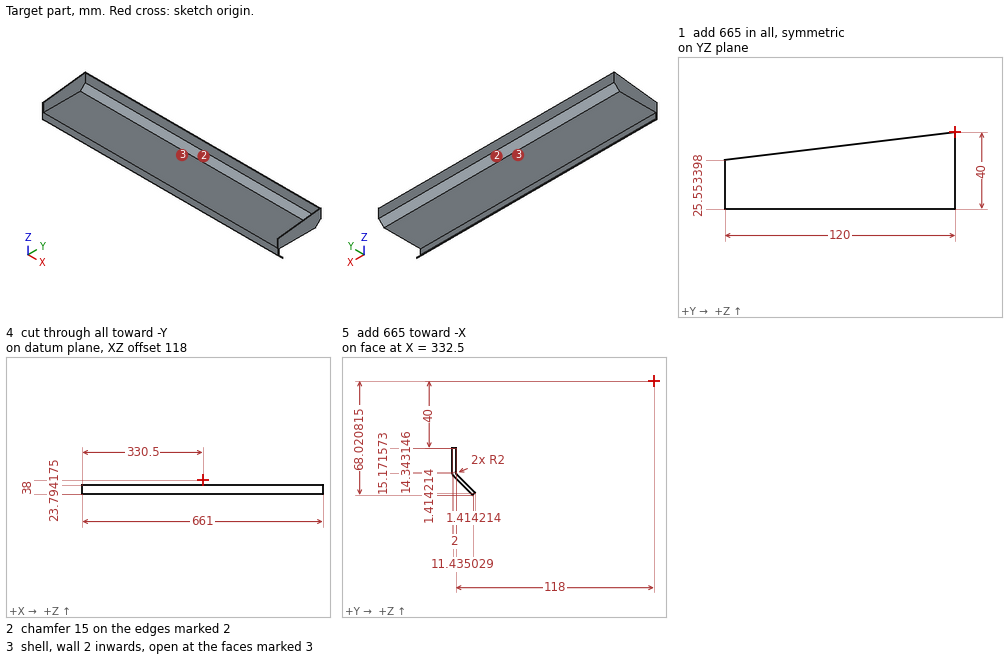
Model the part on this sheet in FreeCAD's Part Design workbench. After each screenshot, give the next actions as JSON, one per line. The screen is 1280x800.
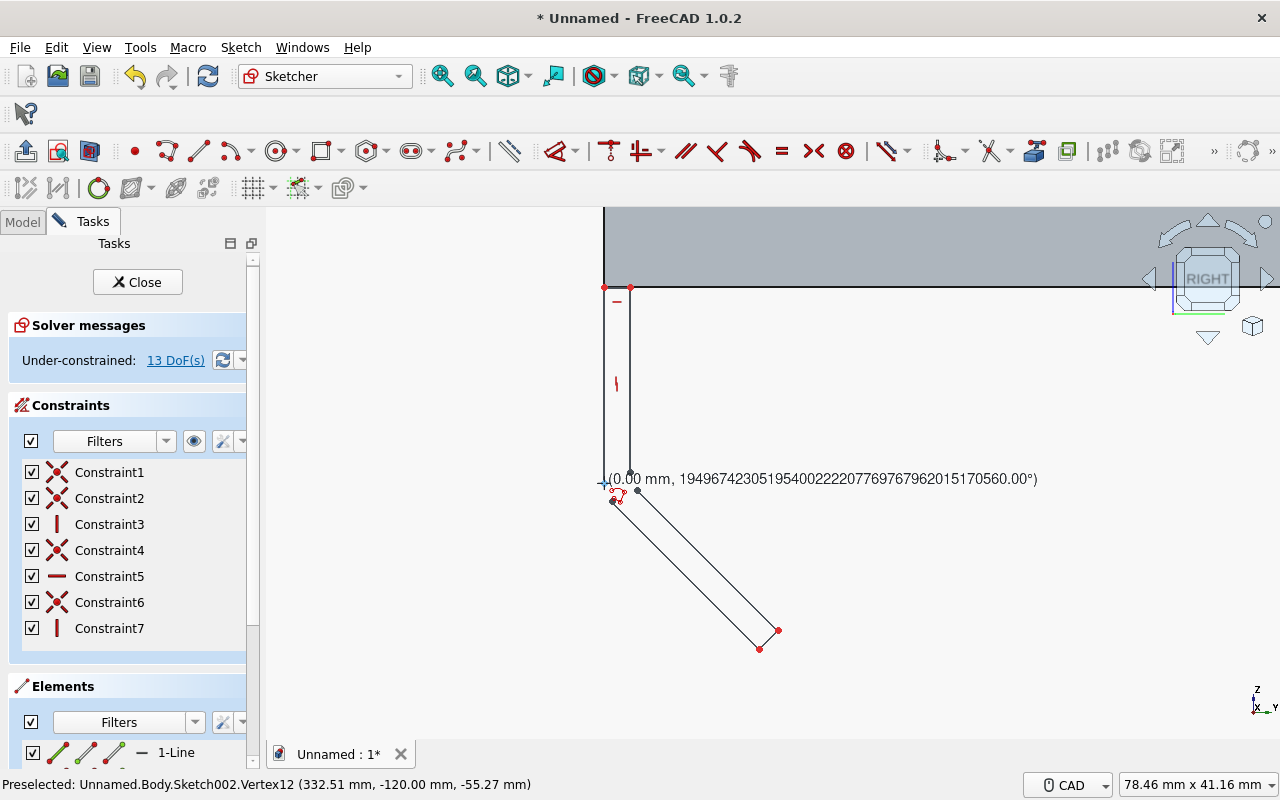
{"action": "key", "text": "g 3 a"}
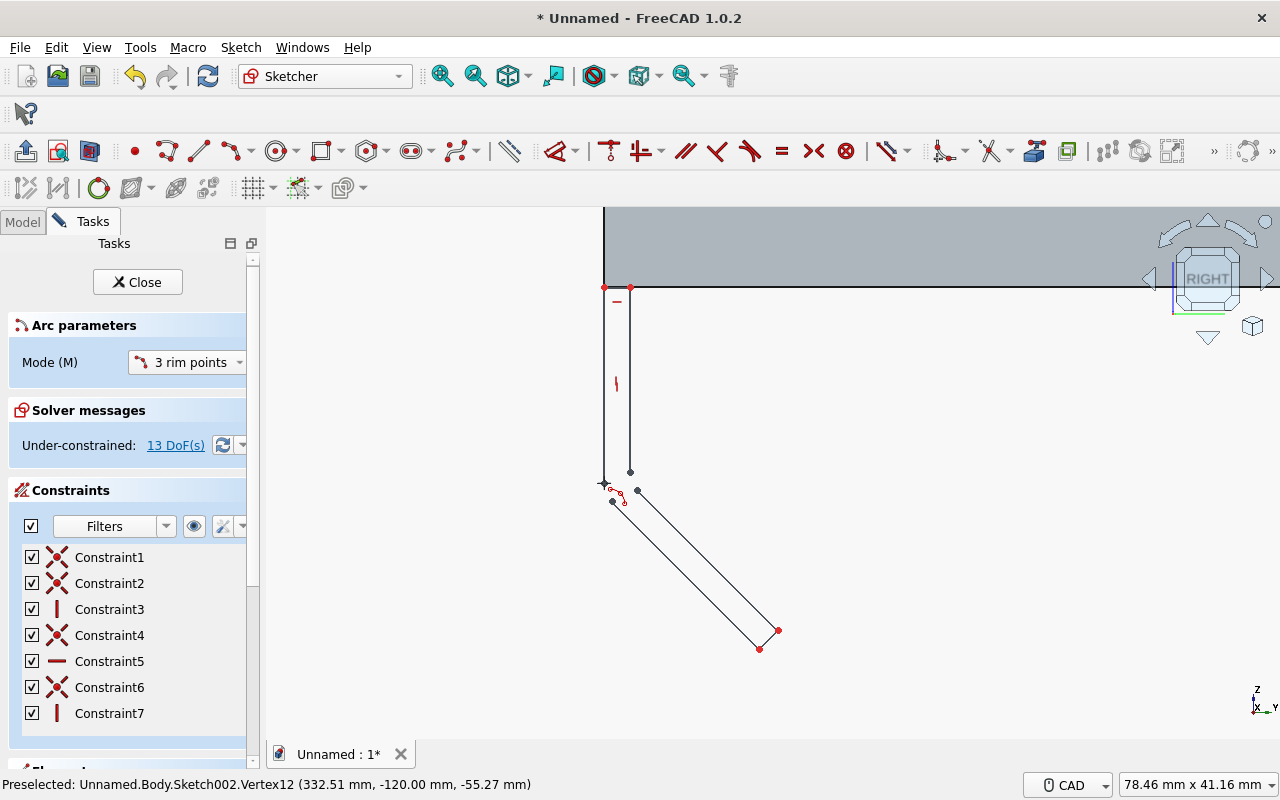
{"action": "left_click", "coordinate": [637, 491]}
{"action": "left_click", "coordinate": [630, 473]}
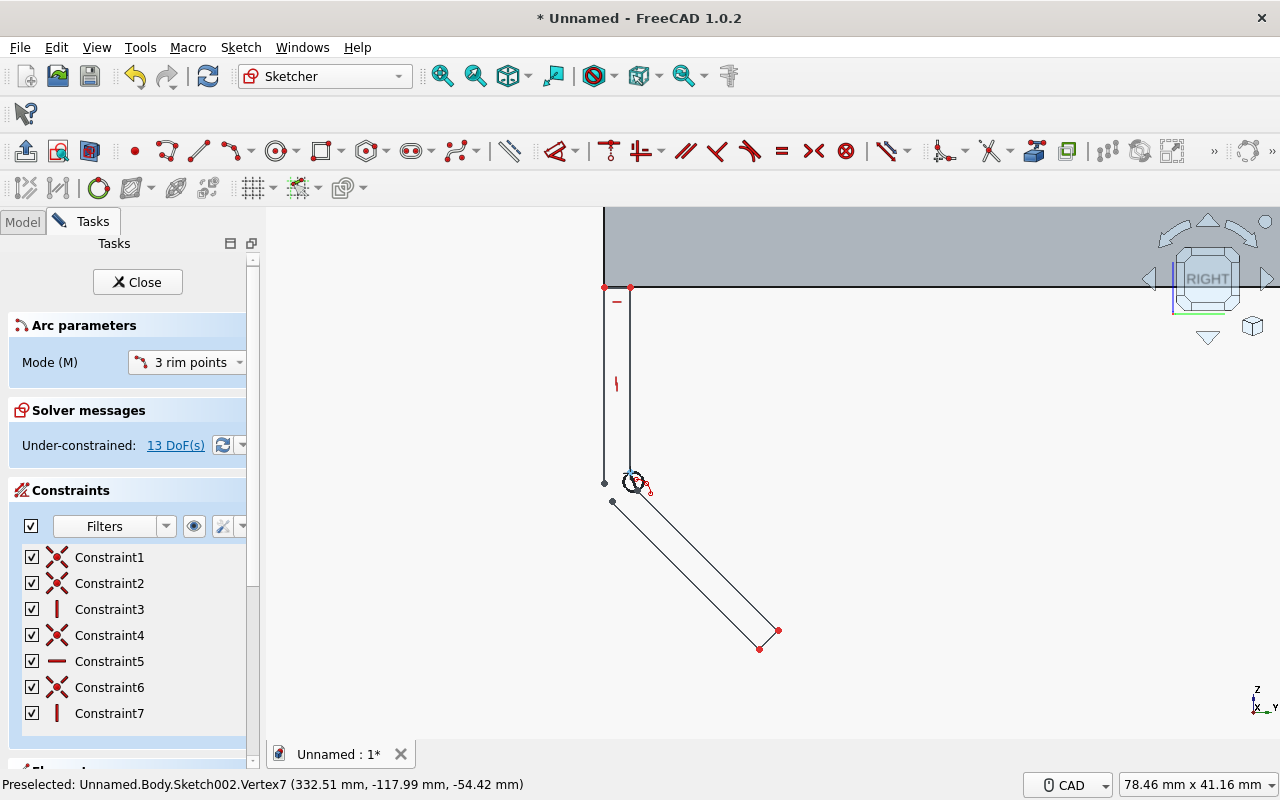
{"action": "scroll", "coordinate": [632, 482], "scroll_direction": "up", "scroll_amount": 11}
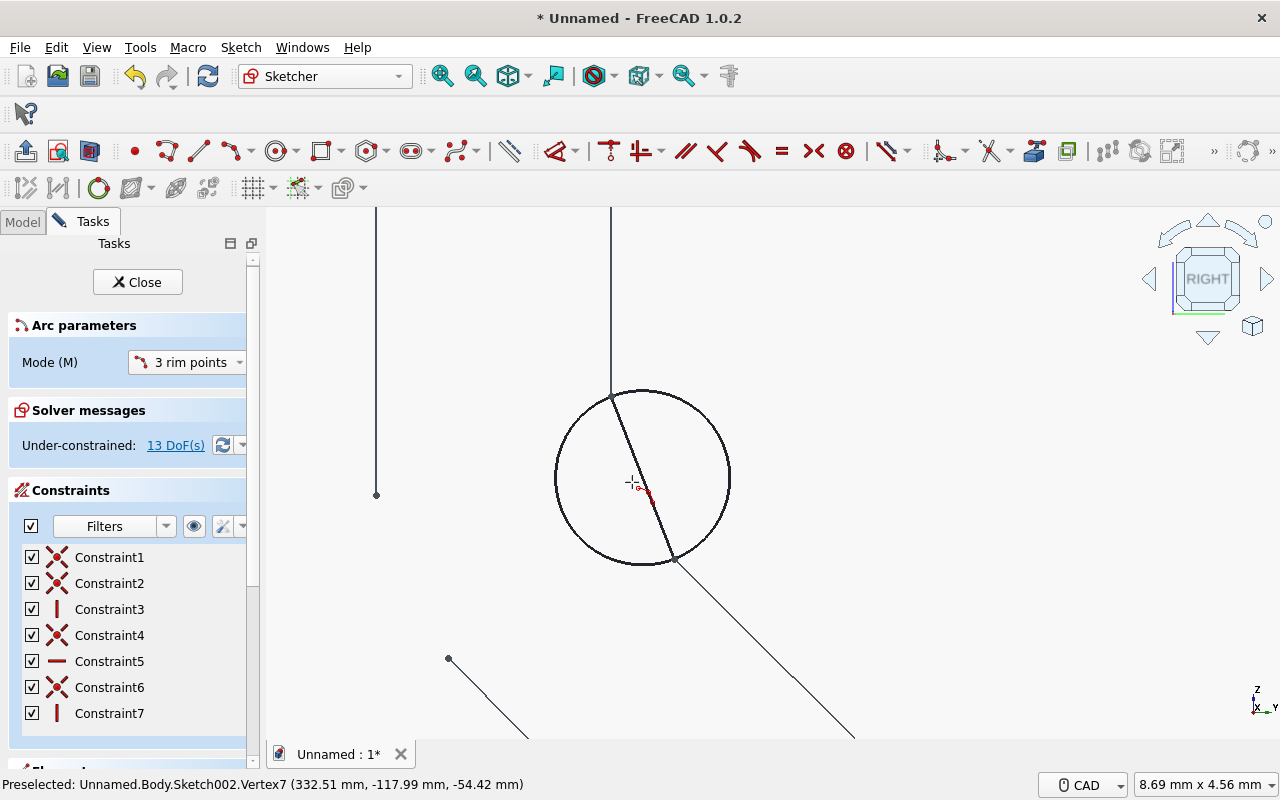
{"action": "left_click", "coordinate": [627, 476]}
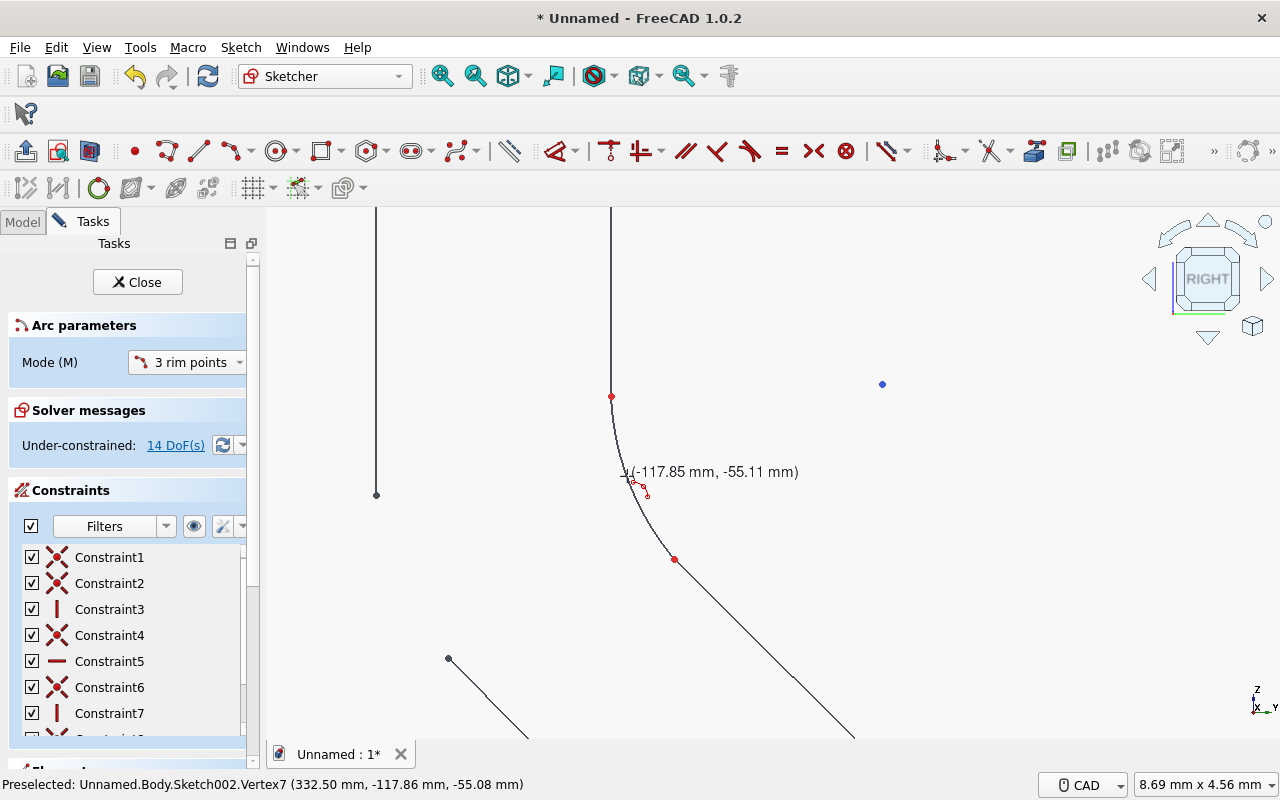
{"action": "scroll", "coordinate": [648, 489], "scroll_direction": "down", "scroll_amount": 11}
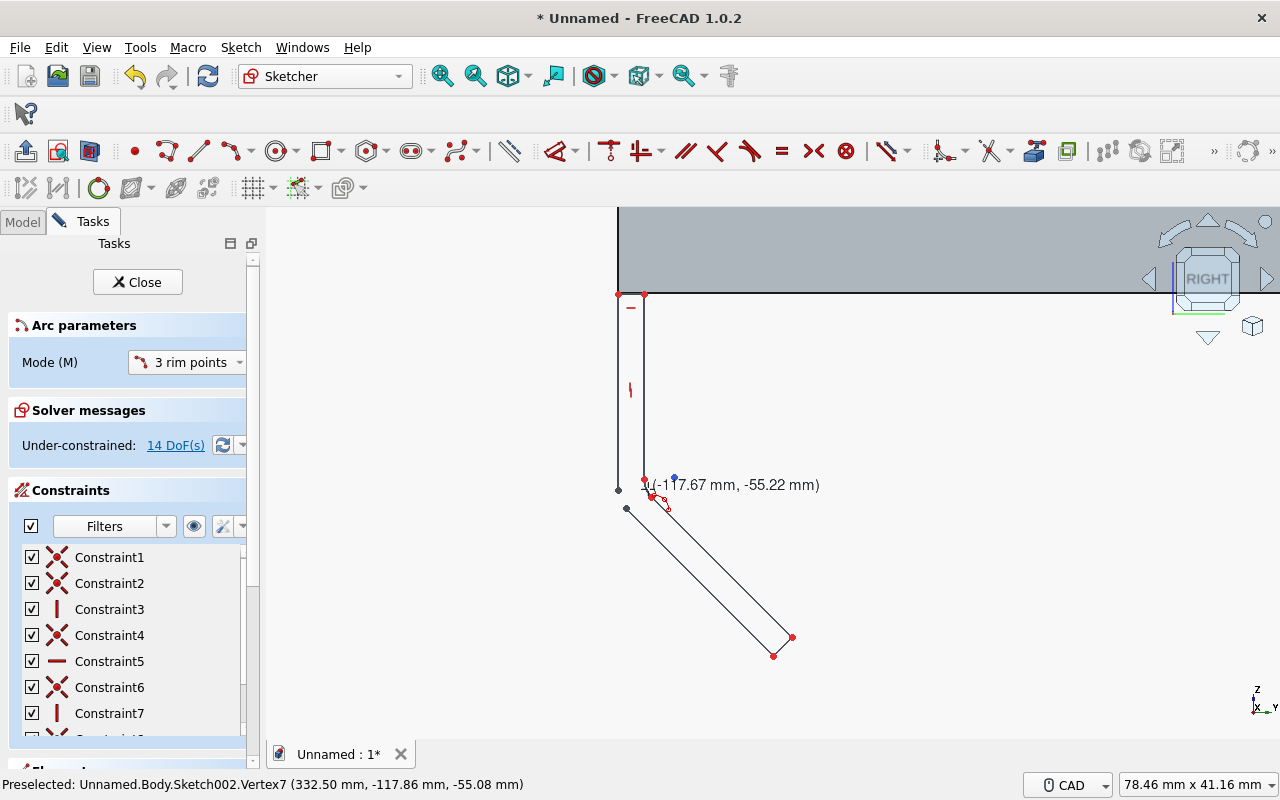
{"action": "left_click", "coordinate": [618, 490]}
{"action": "left_click", "coordinate": [626, 508]}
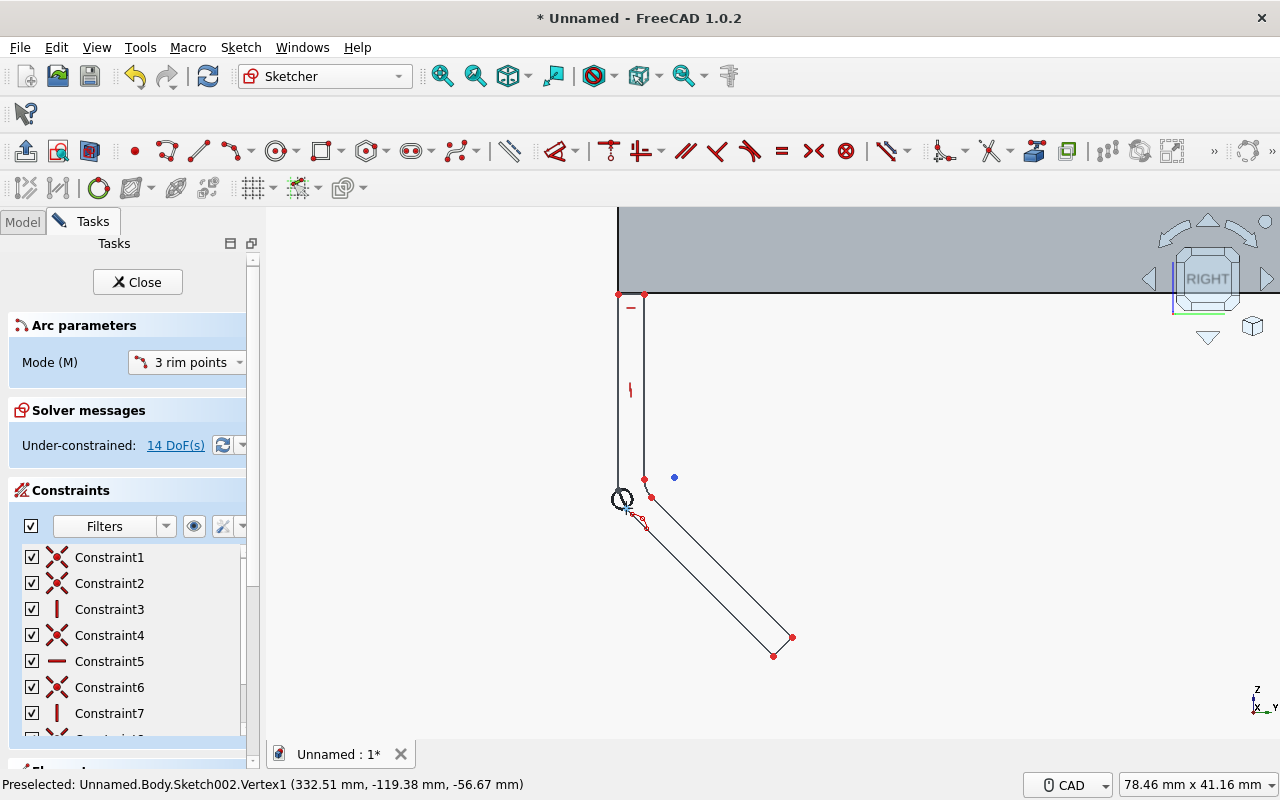
{"action": "scroll", "coordinate": [620, 499], "scroll_direction": "up", "scroll_amount": 11}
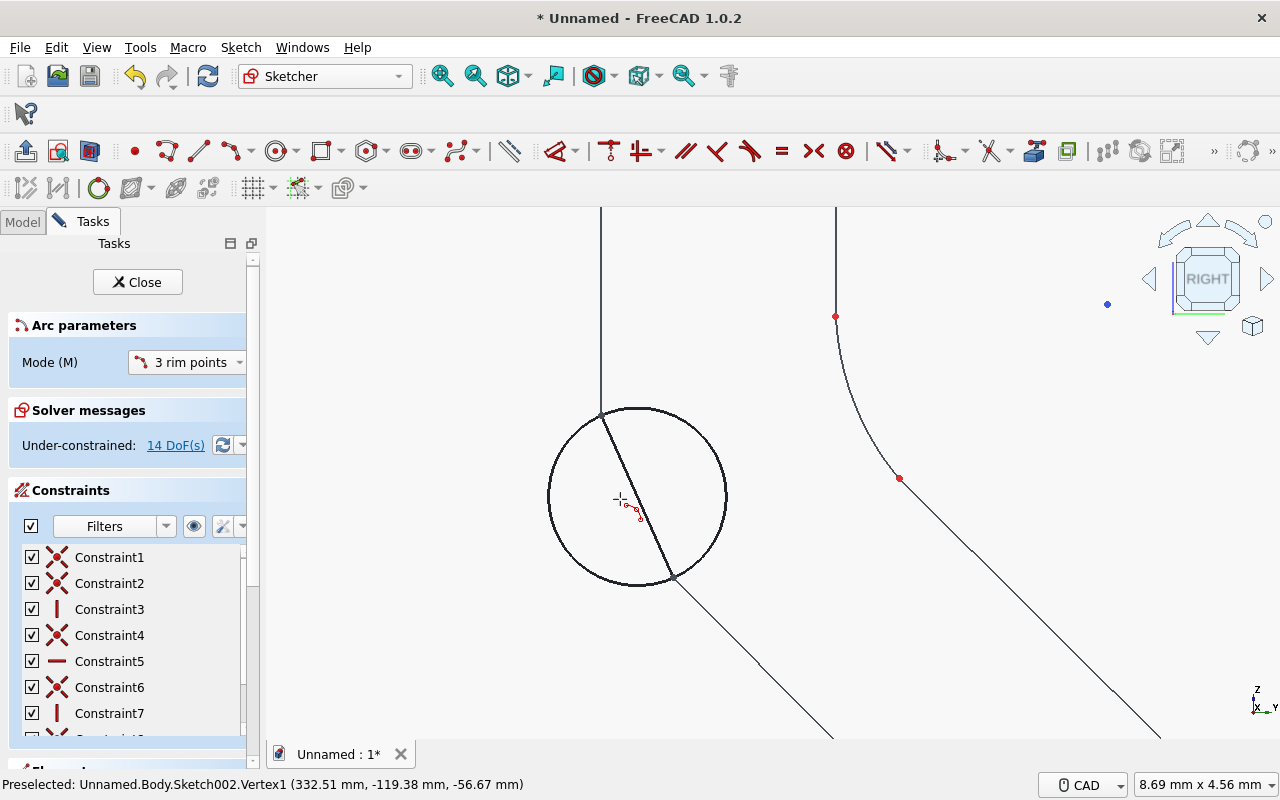
{"action": "left_click", "coordinate": [619, 493]}
{"action": "key", "text": "Escape"}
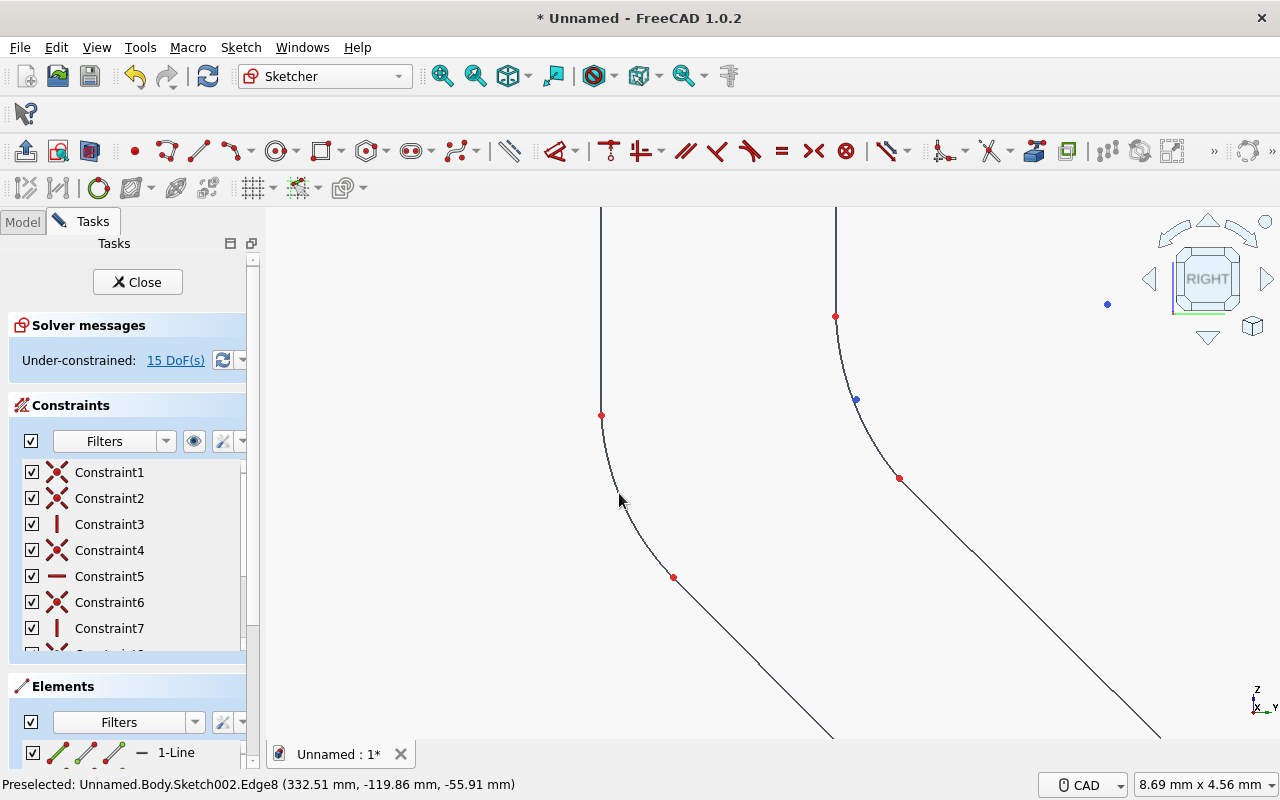
{"action": "scroll", "coordinate": [620, 499], "scroll_direction": "down", "scroll_amount": 11}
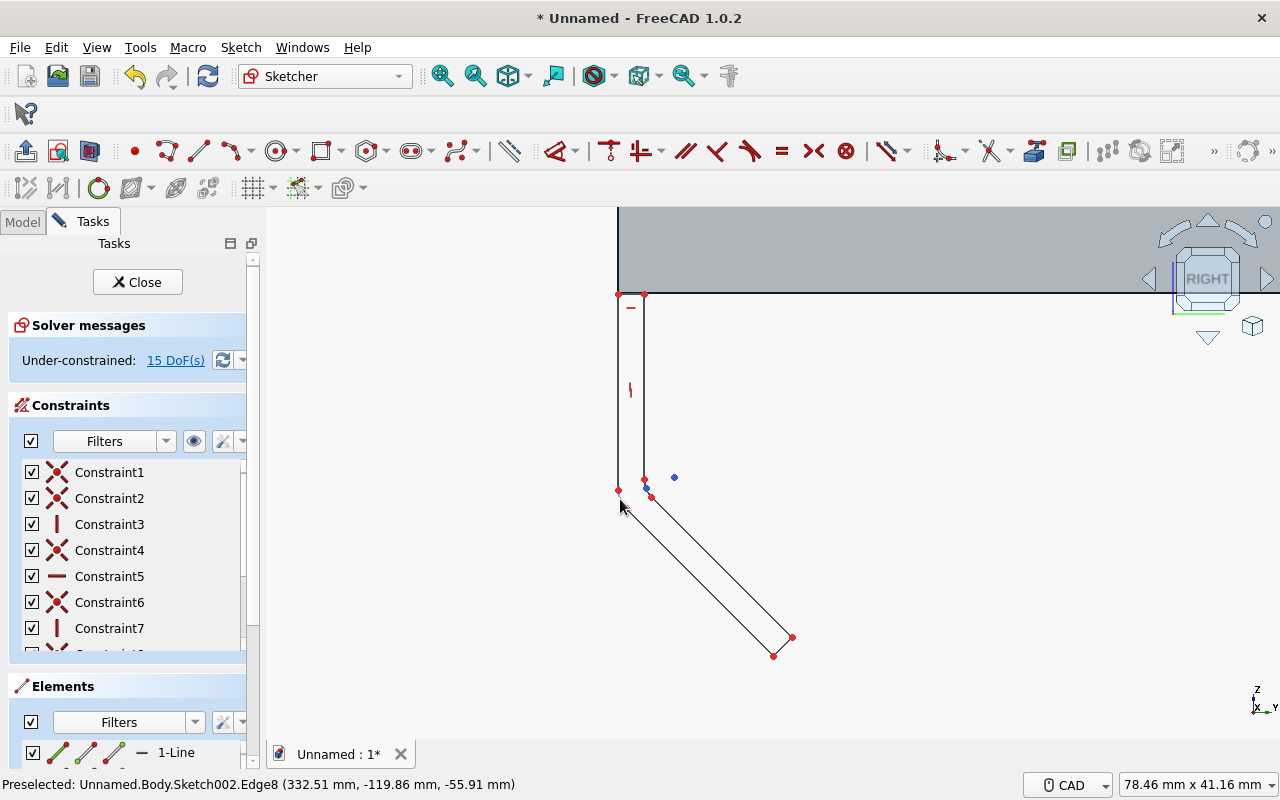
{"action": "left_click", "coordinate": [670, 553]}